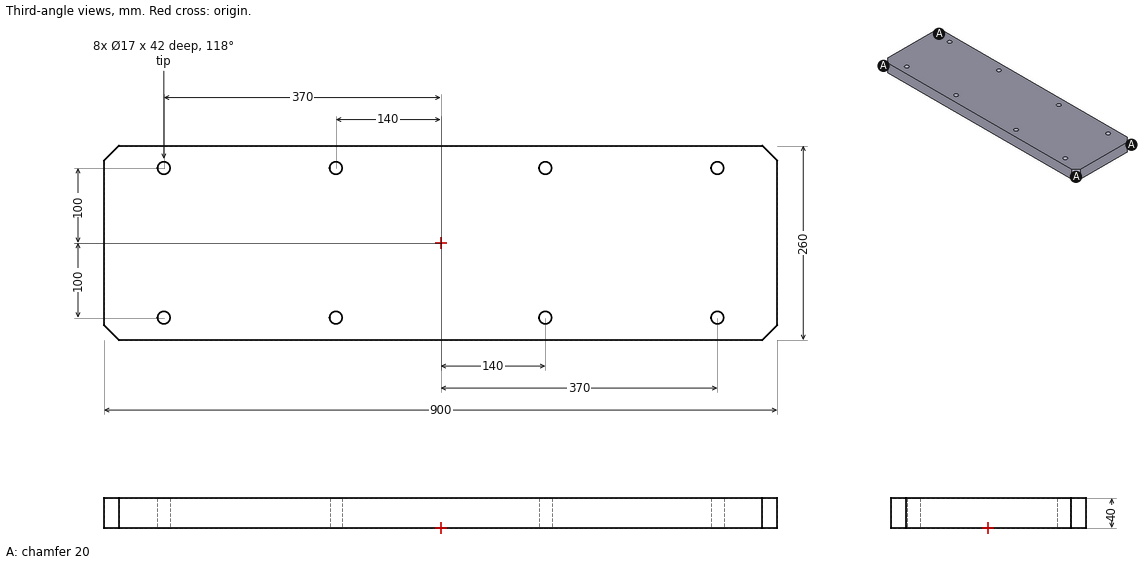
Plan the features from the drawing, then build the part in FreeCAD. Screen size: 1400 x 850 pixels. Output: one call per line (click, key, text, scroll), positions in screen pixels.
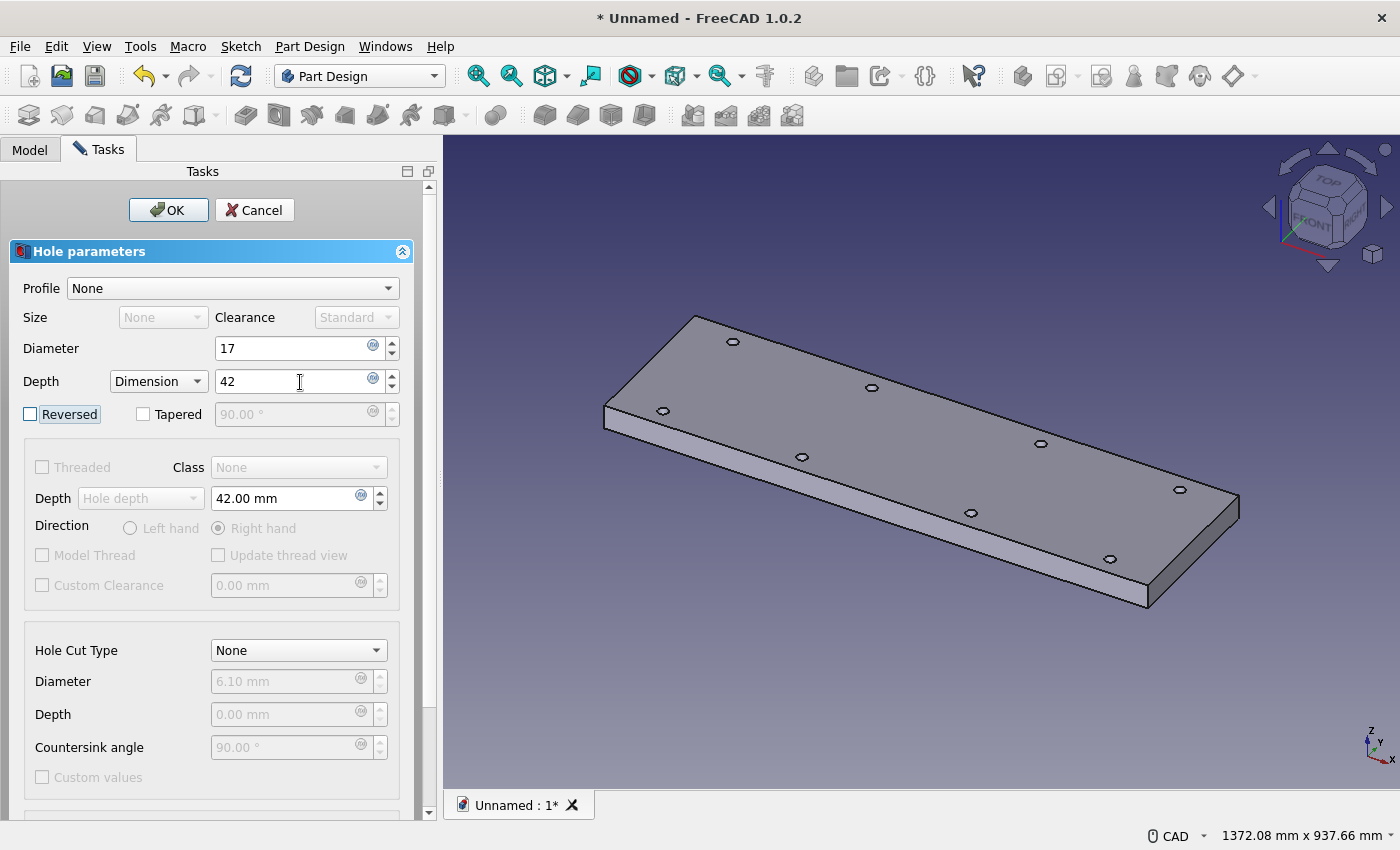
click(169, 210)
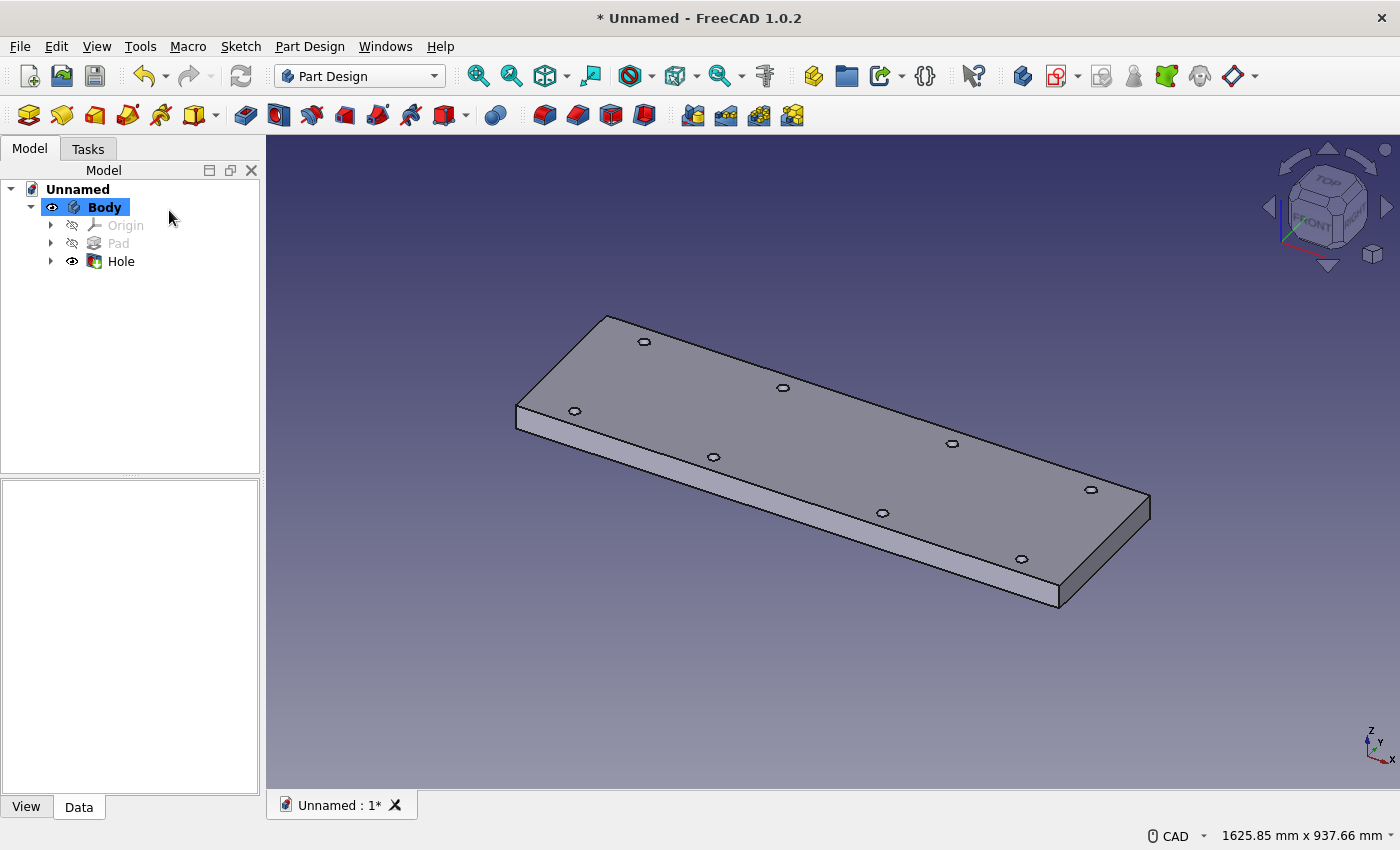
click(1059, 596)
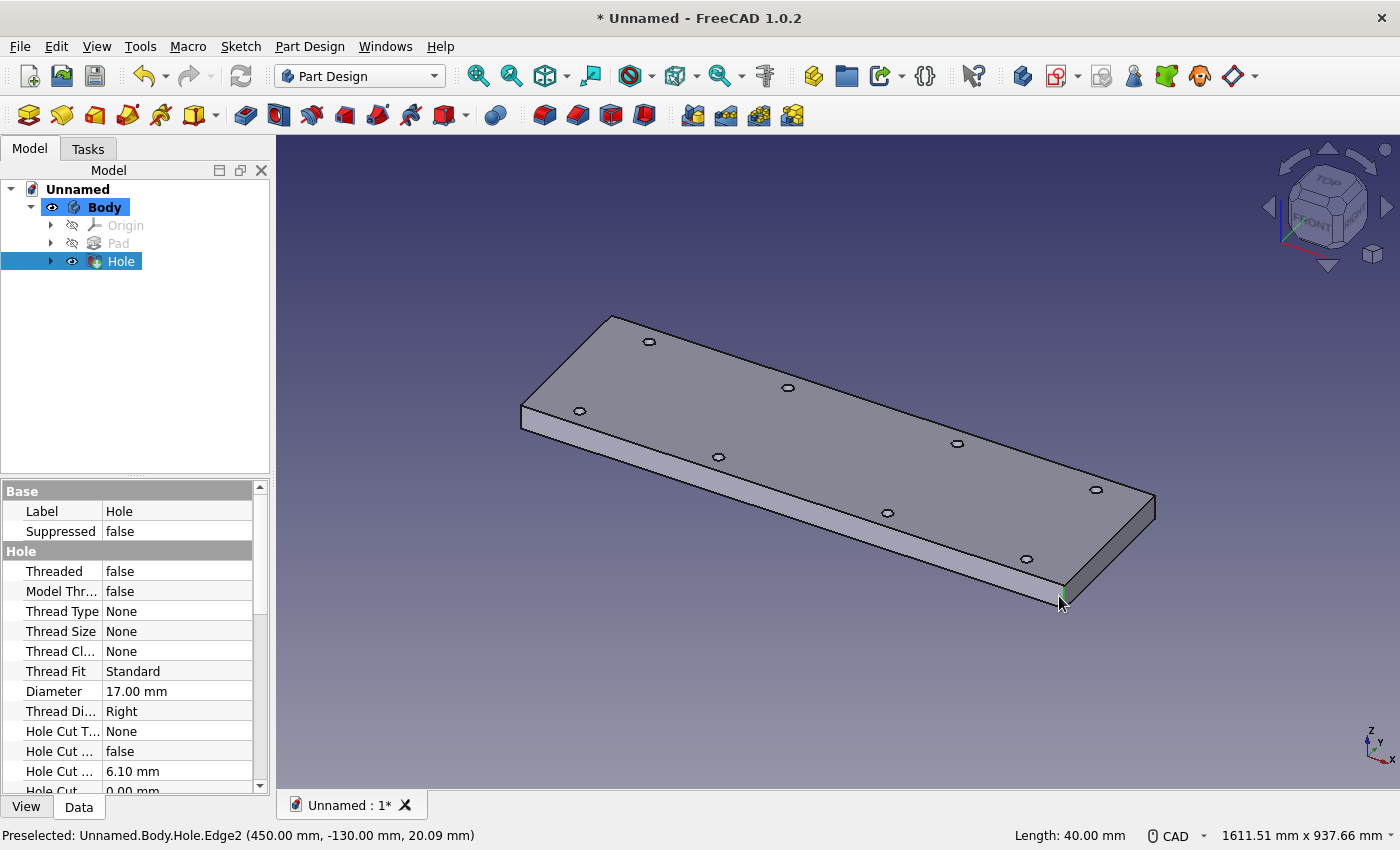
key(0)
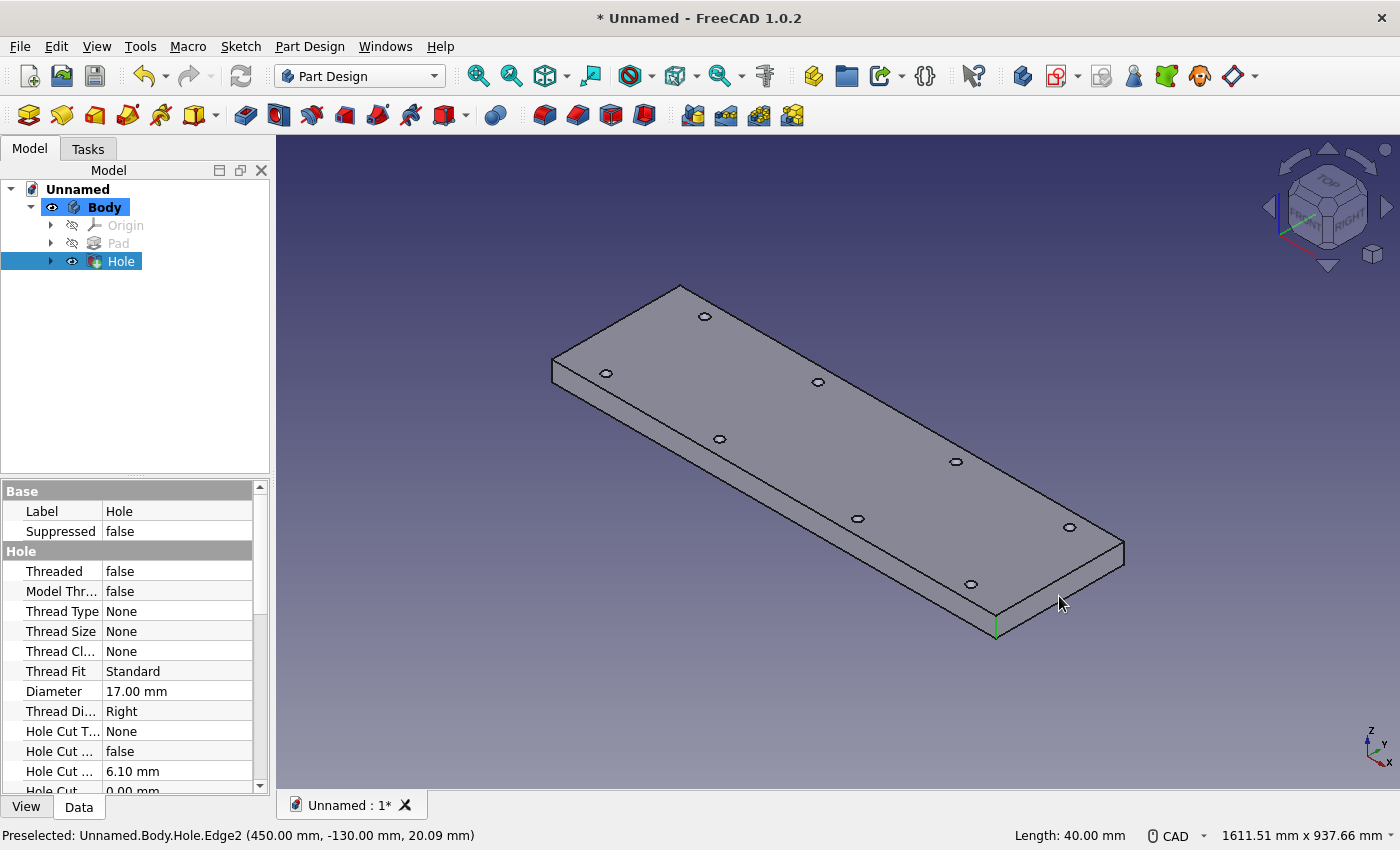
key(2)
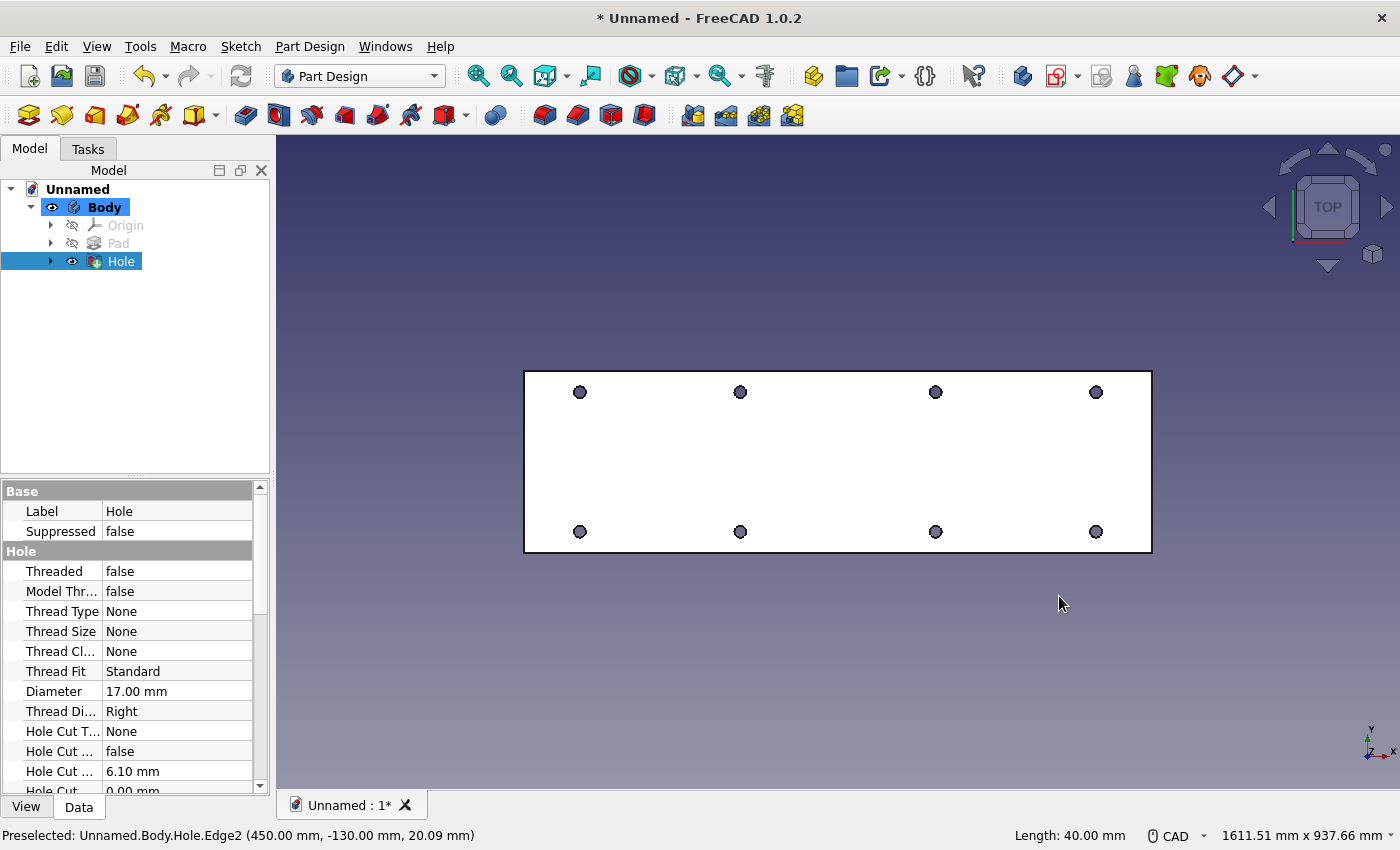
key(1)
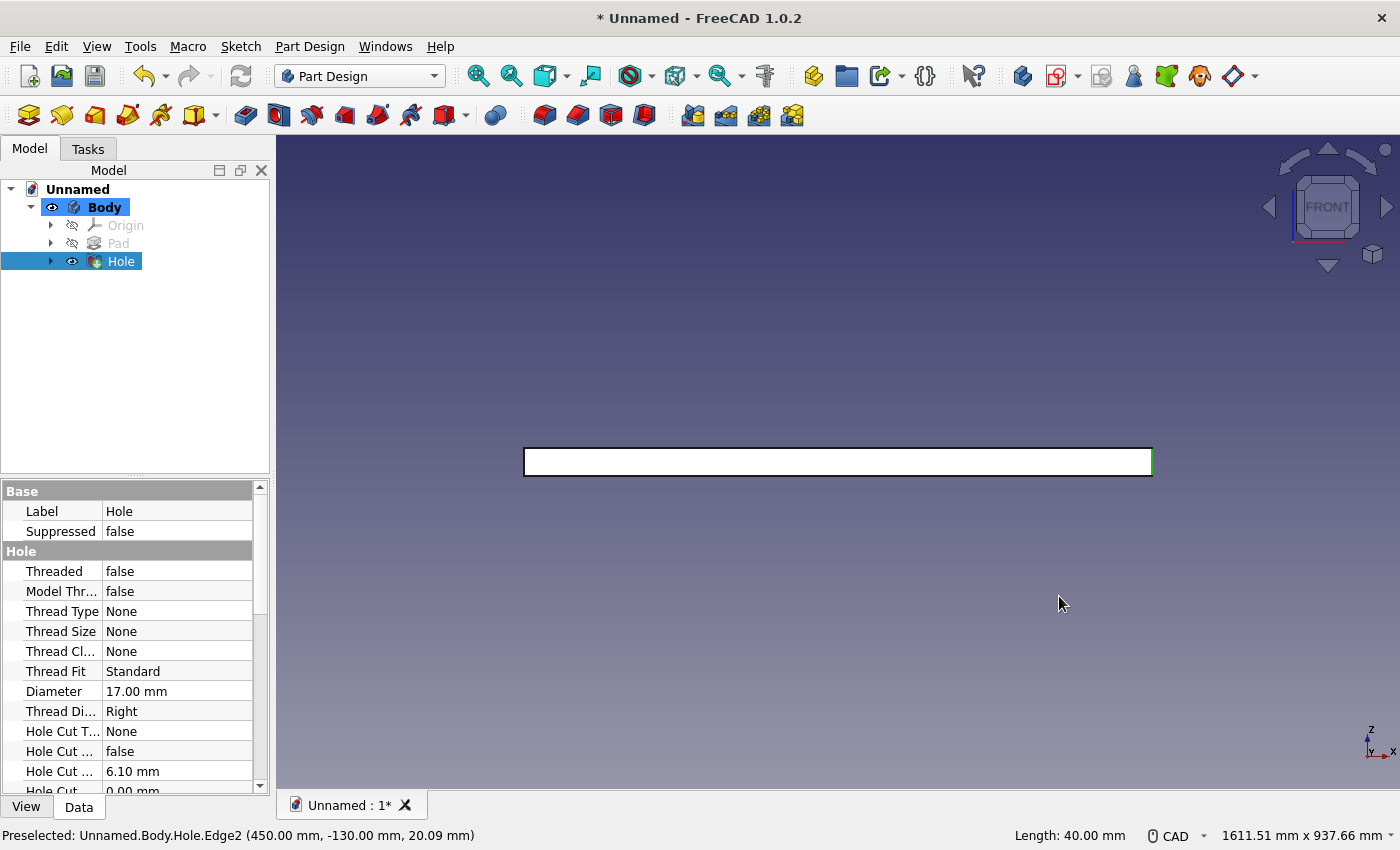
click(524, 461, ctrl)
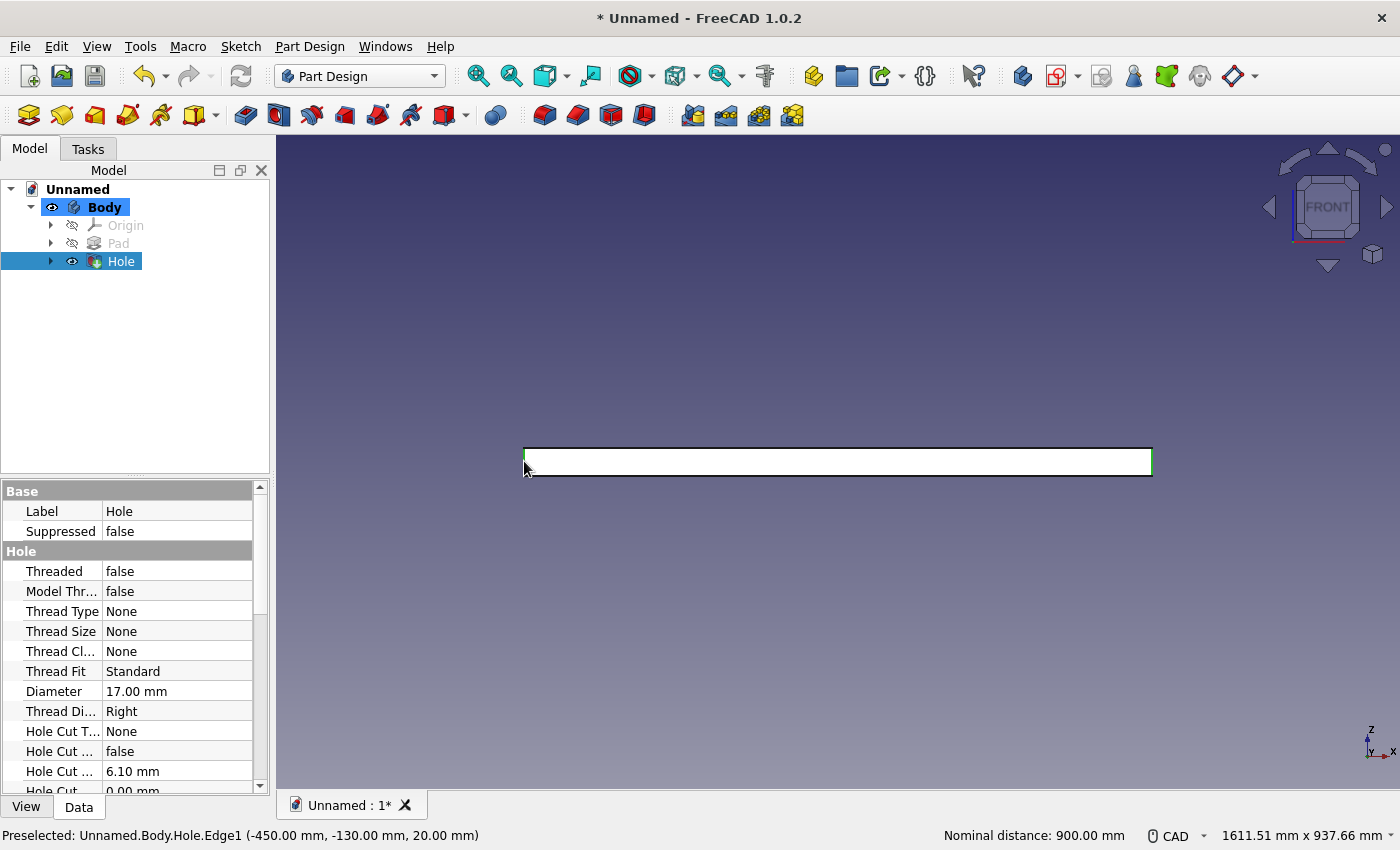
key(3)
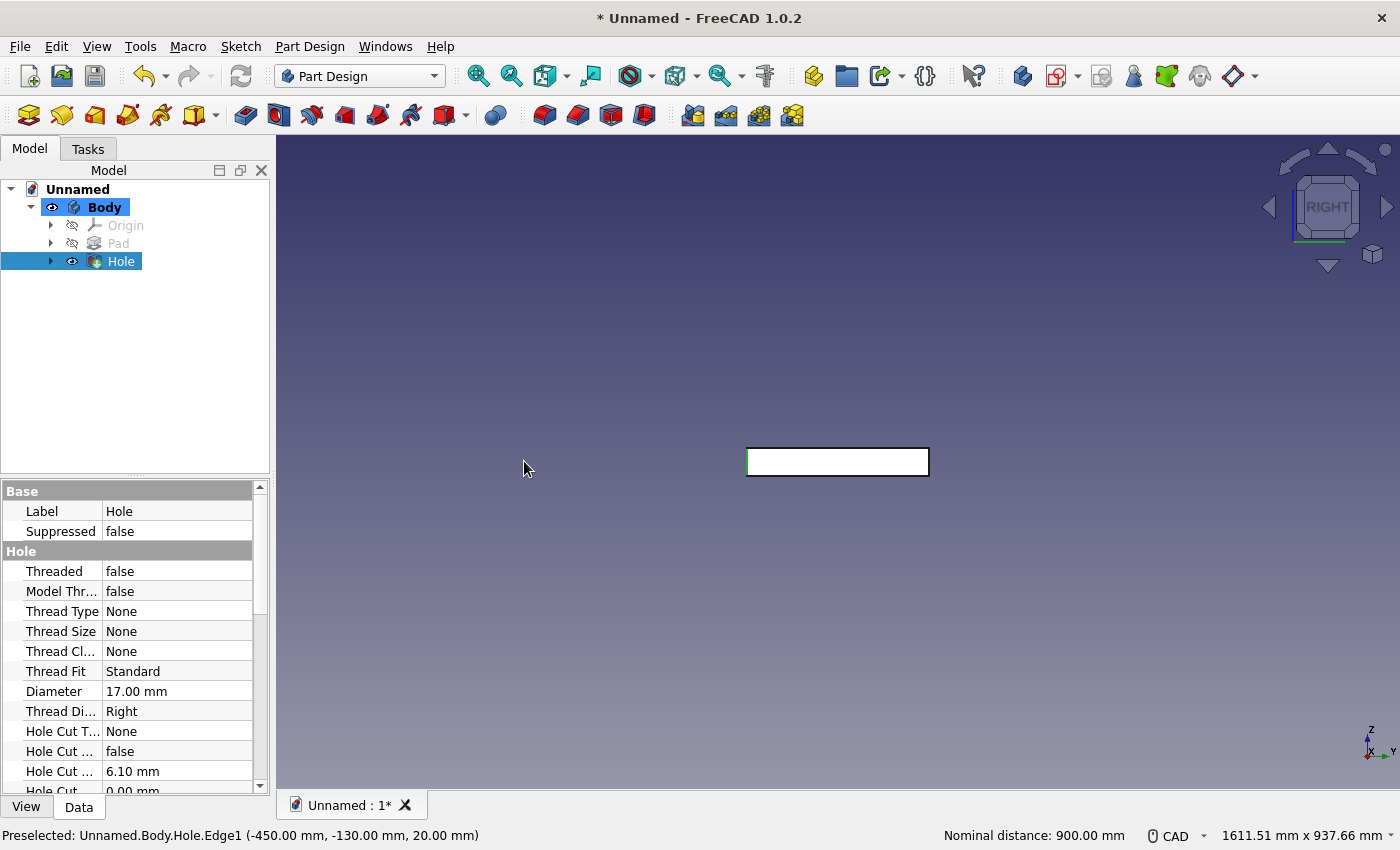
click(479, 76)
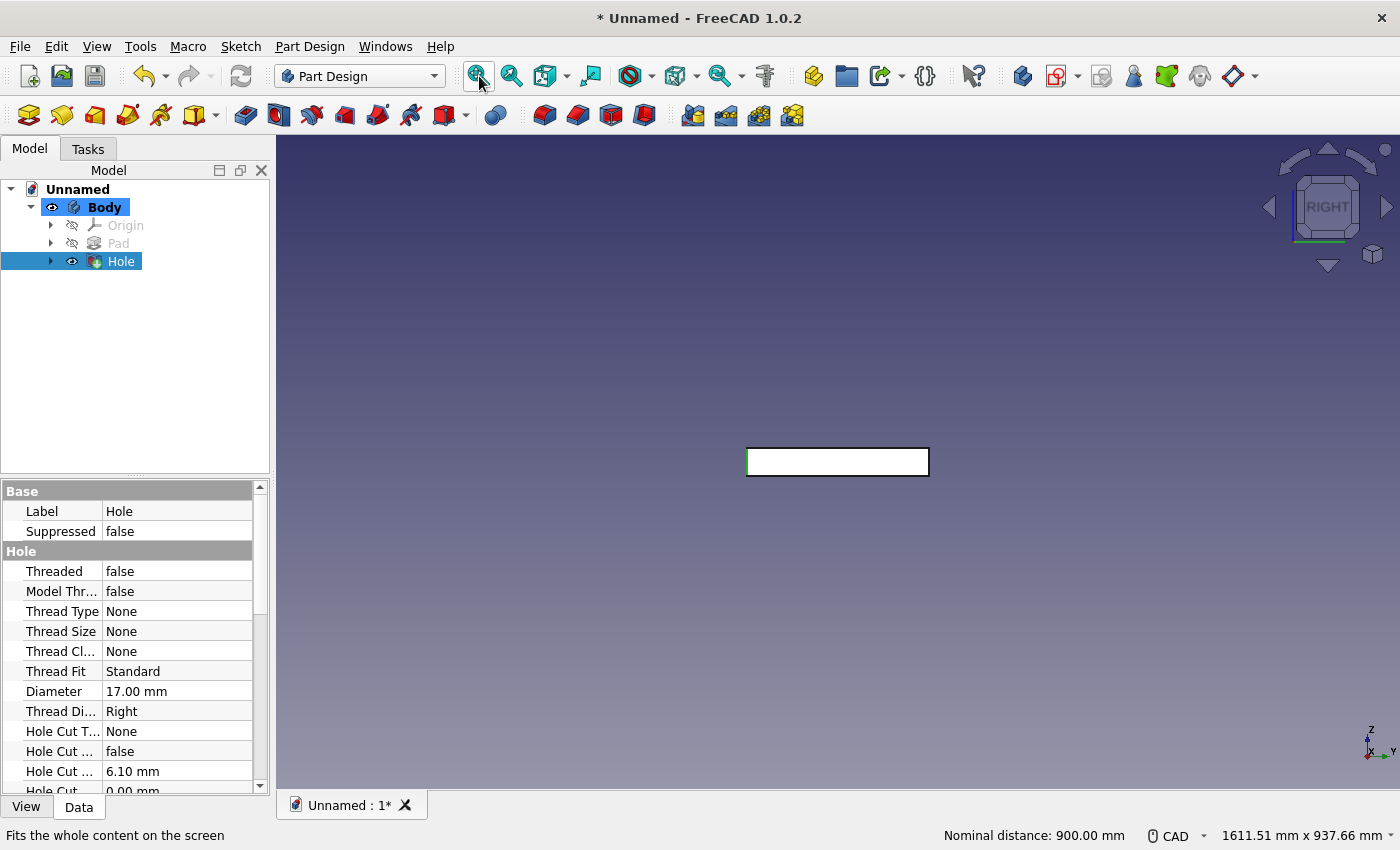
click(929, 461, ctrl)